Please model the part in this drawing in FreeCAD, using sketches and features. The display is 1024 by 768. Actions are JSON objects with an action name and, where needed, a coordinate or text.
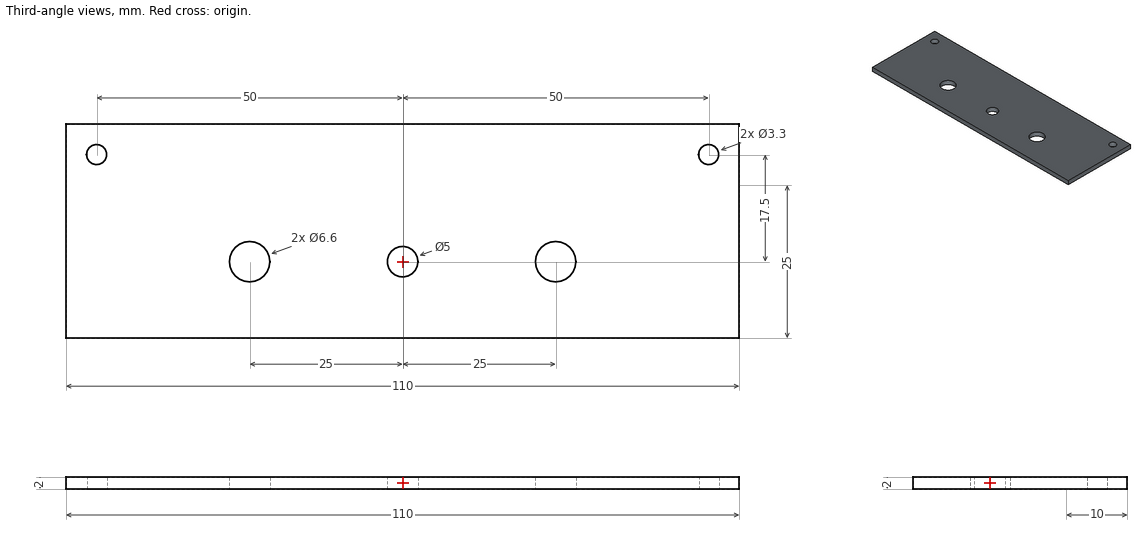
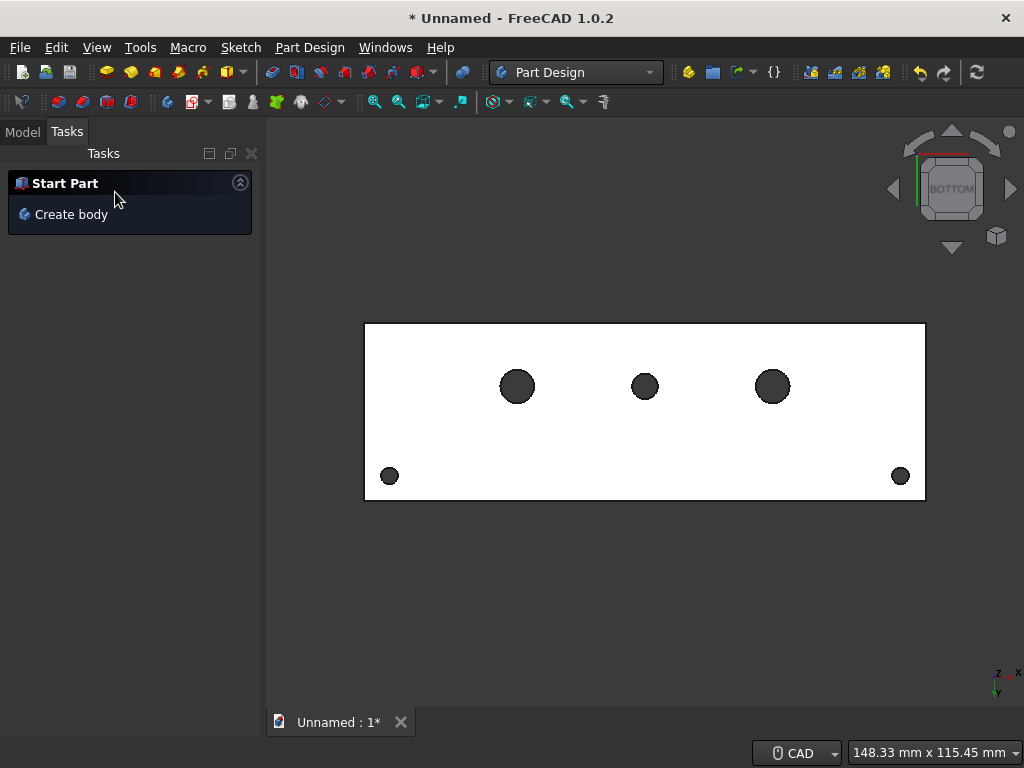
{"action": "key", "text": "0"}